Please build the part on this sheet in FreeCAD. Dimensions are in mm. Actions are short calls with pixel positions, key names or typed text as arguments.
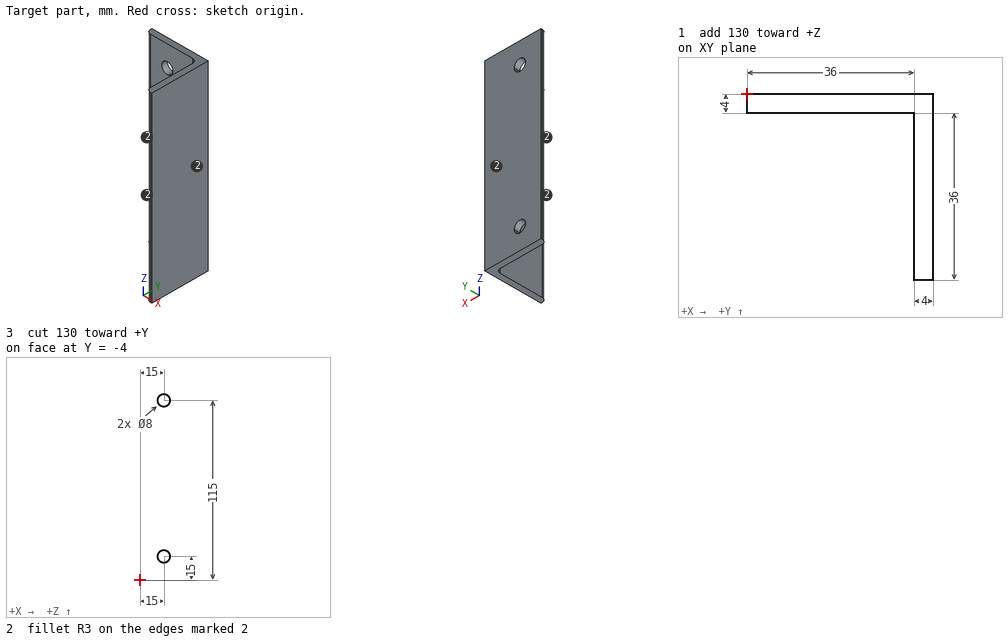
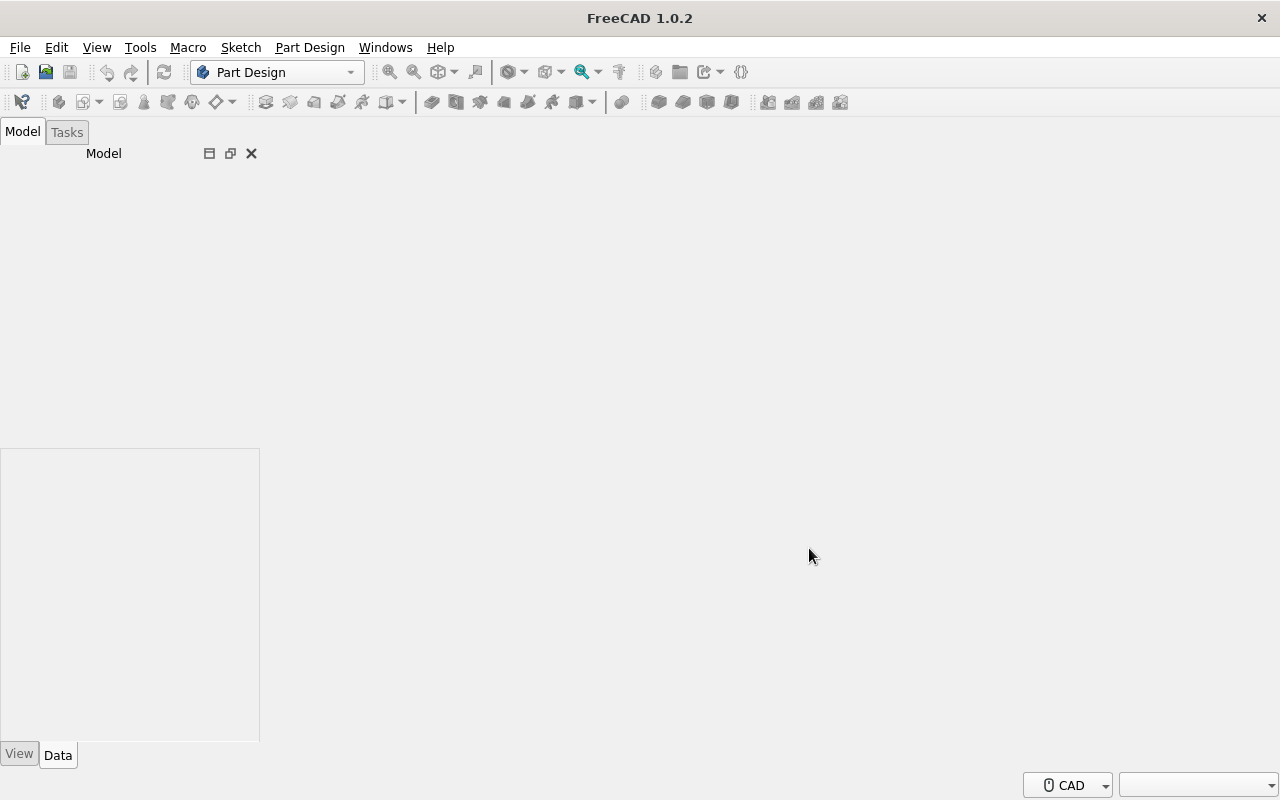
click(22, 72)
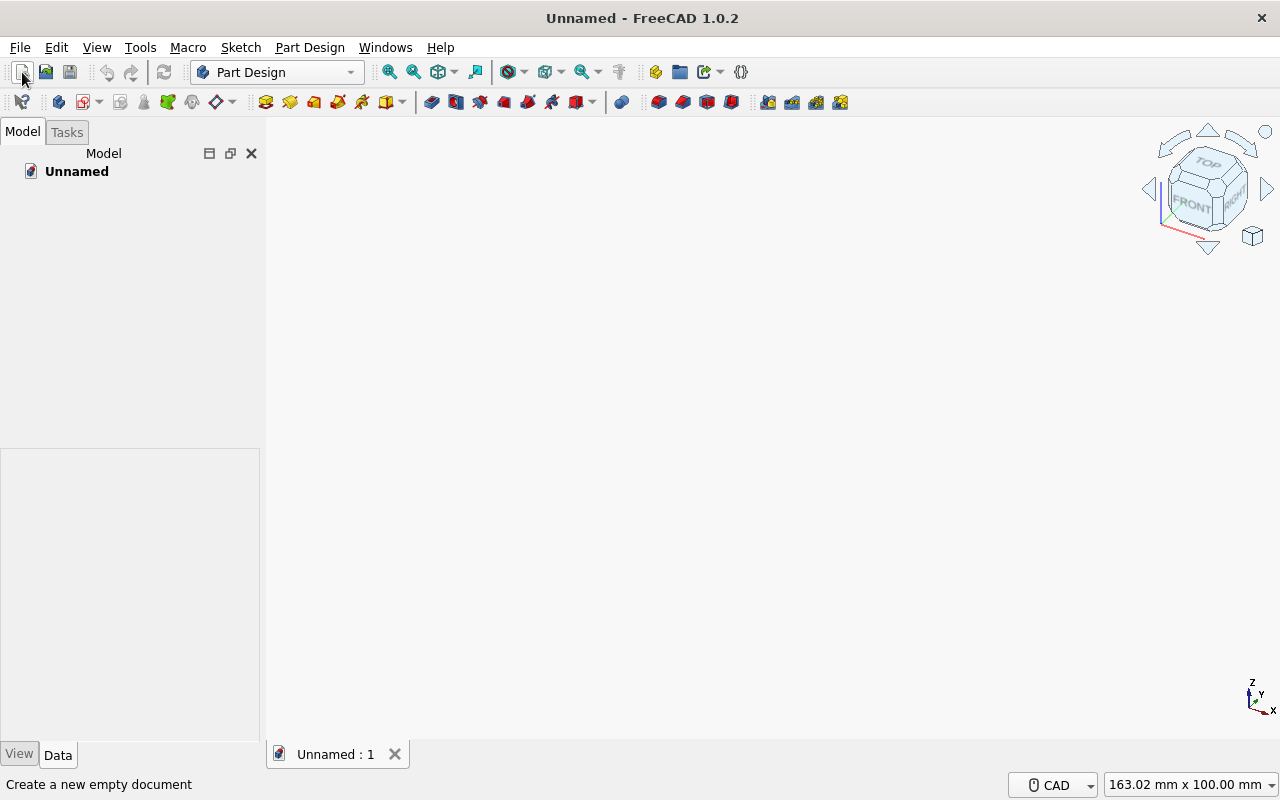
click(84, 102)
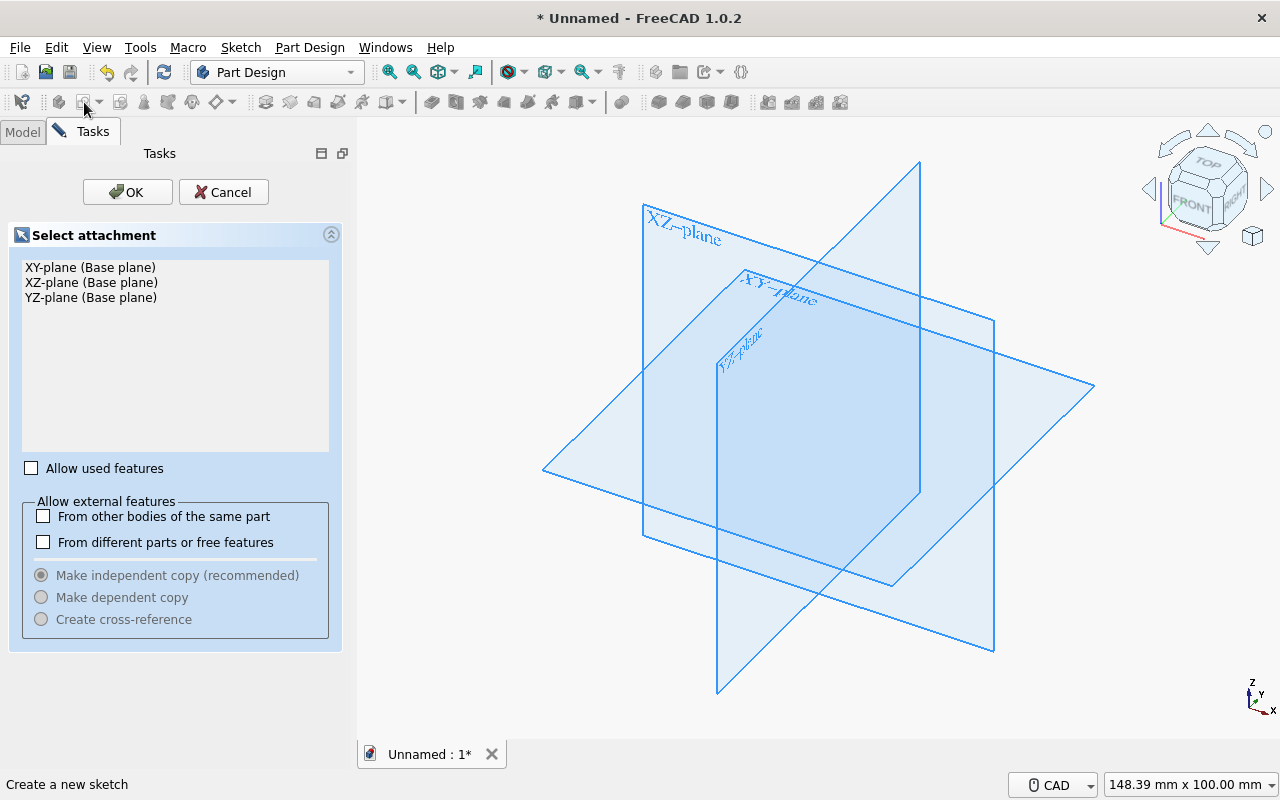
click(82, 268)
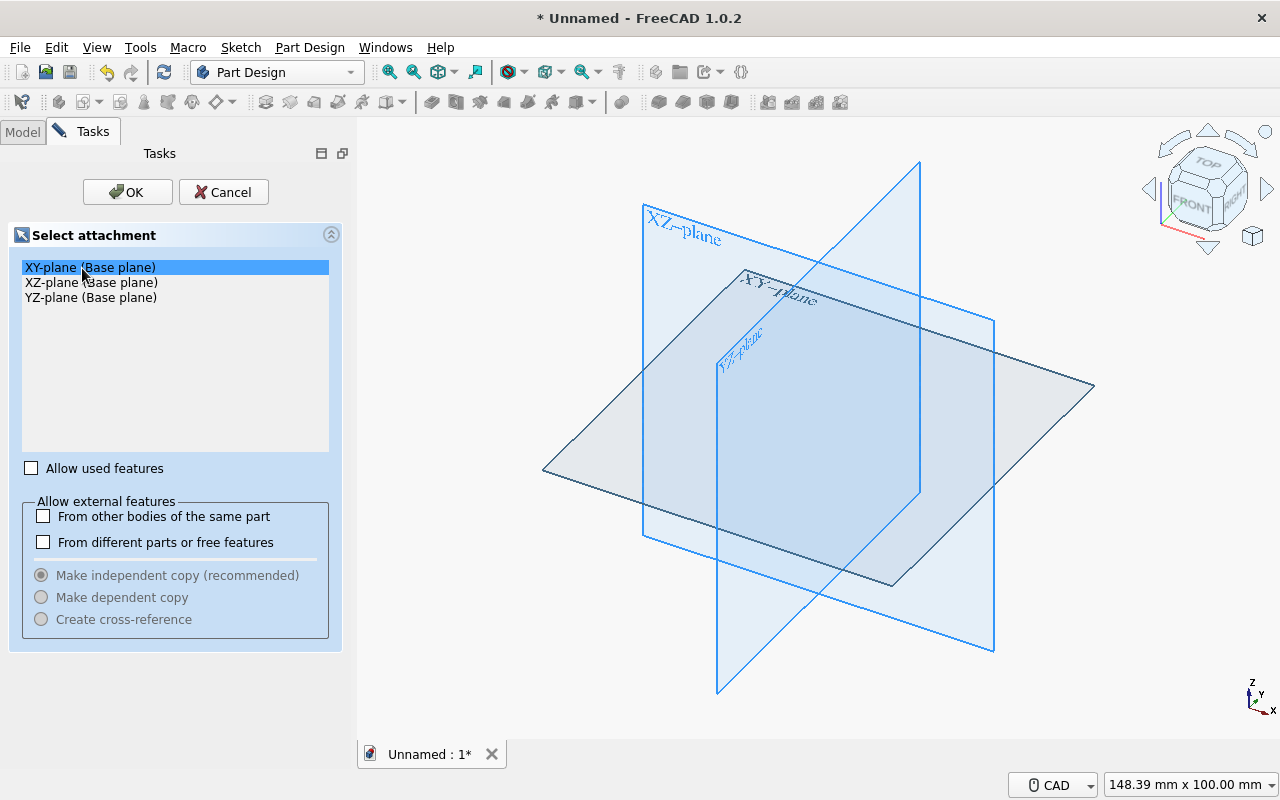
click(128, 192)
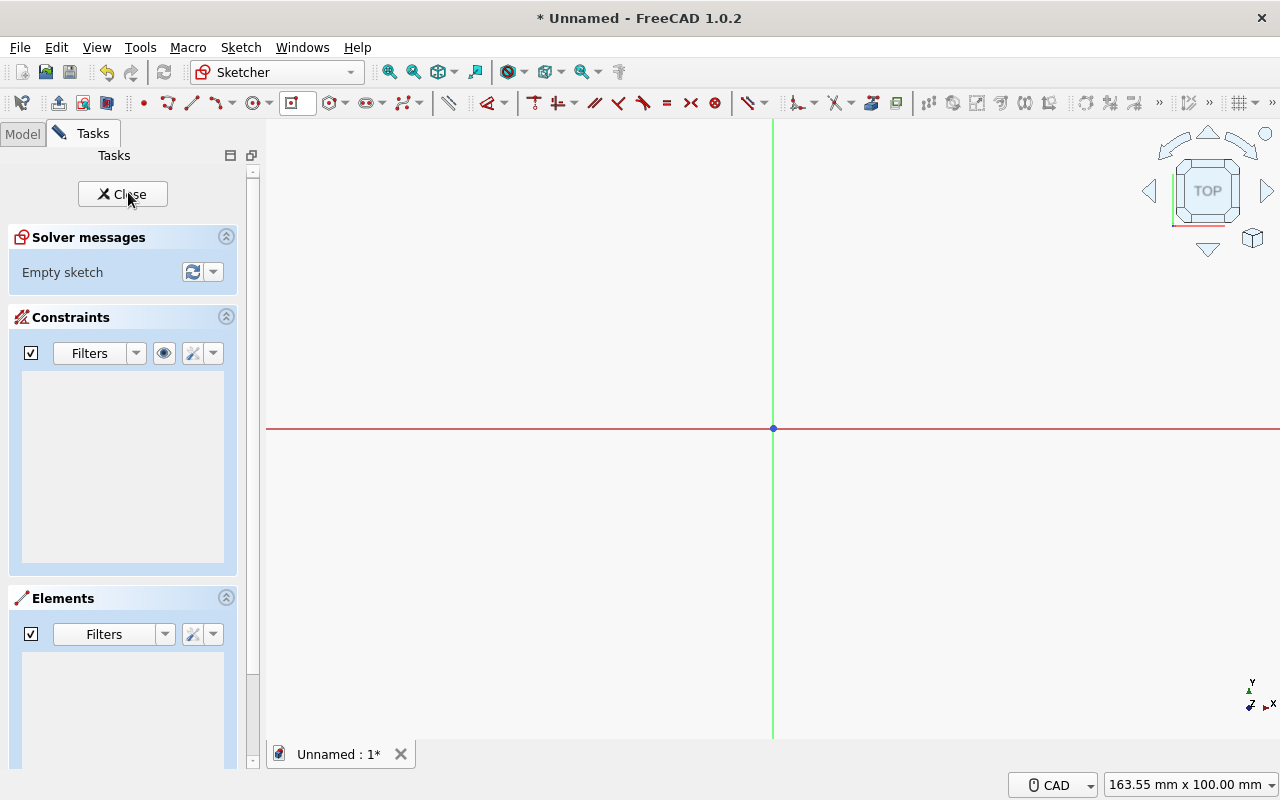
scroll(1115, 711, up, 2)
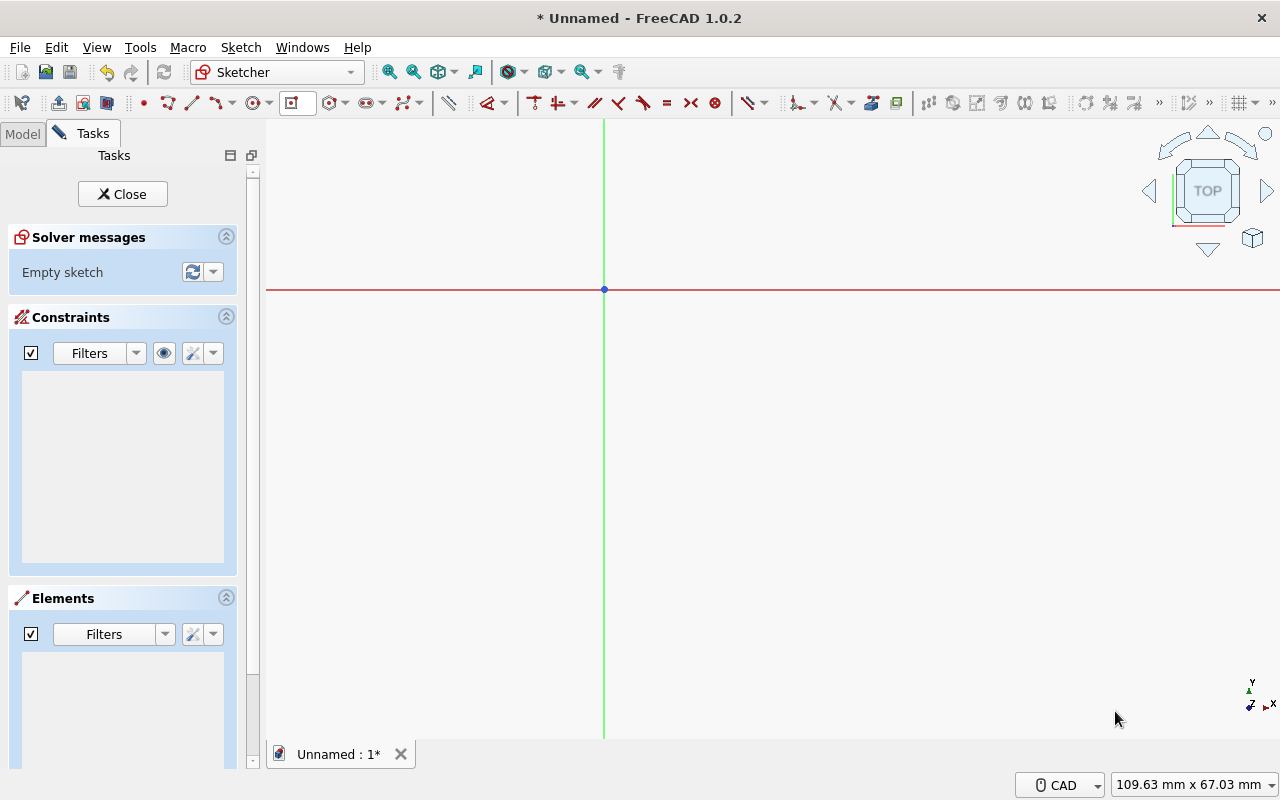
click(168, 104)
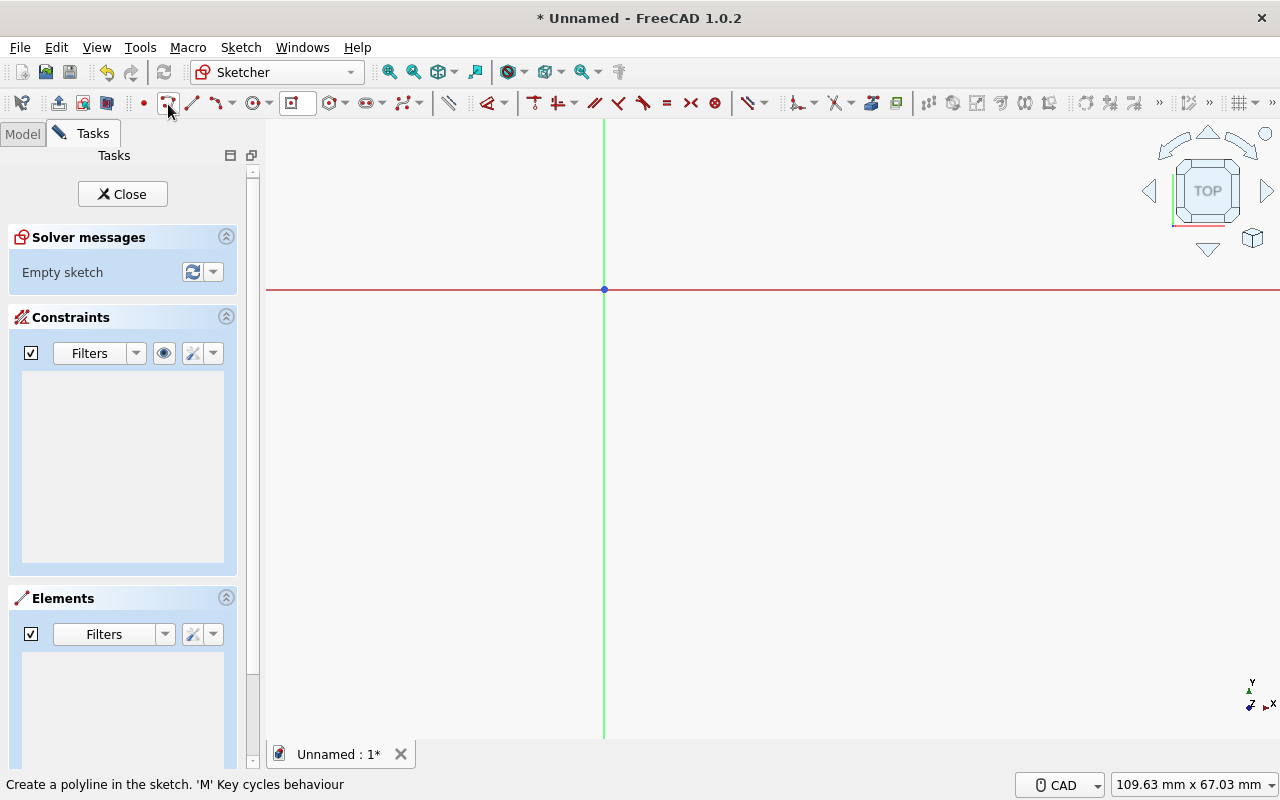
click(604, 290)
click(613, 327)
click(937, 327)
click(937, 660)
click(974, 660)
click(974, 299)
click(604, 290)
key(Escape)
key(Escape)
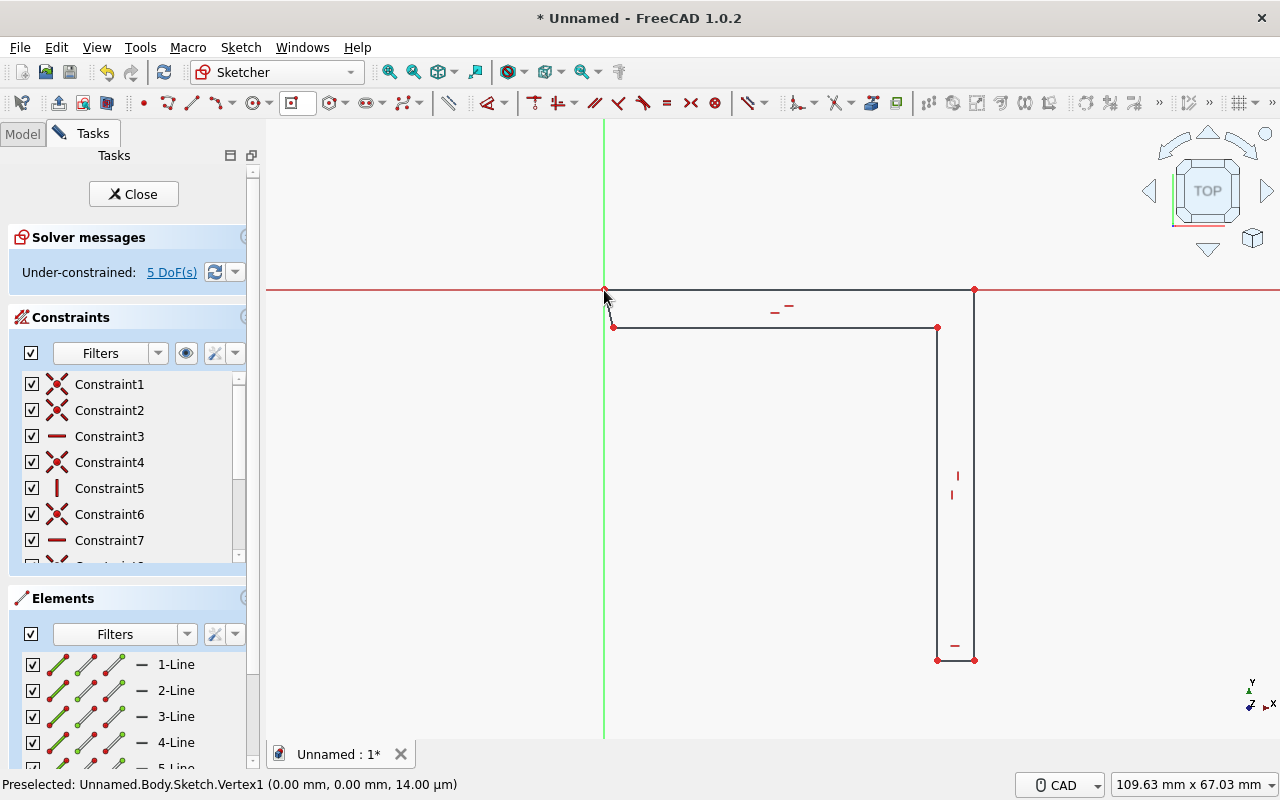
click(607, 301)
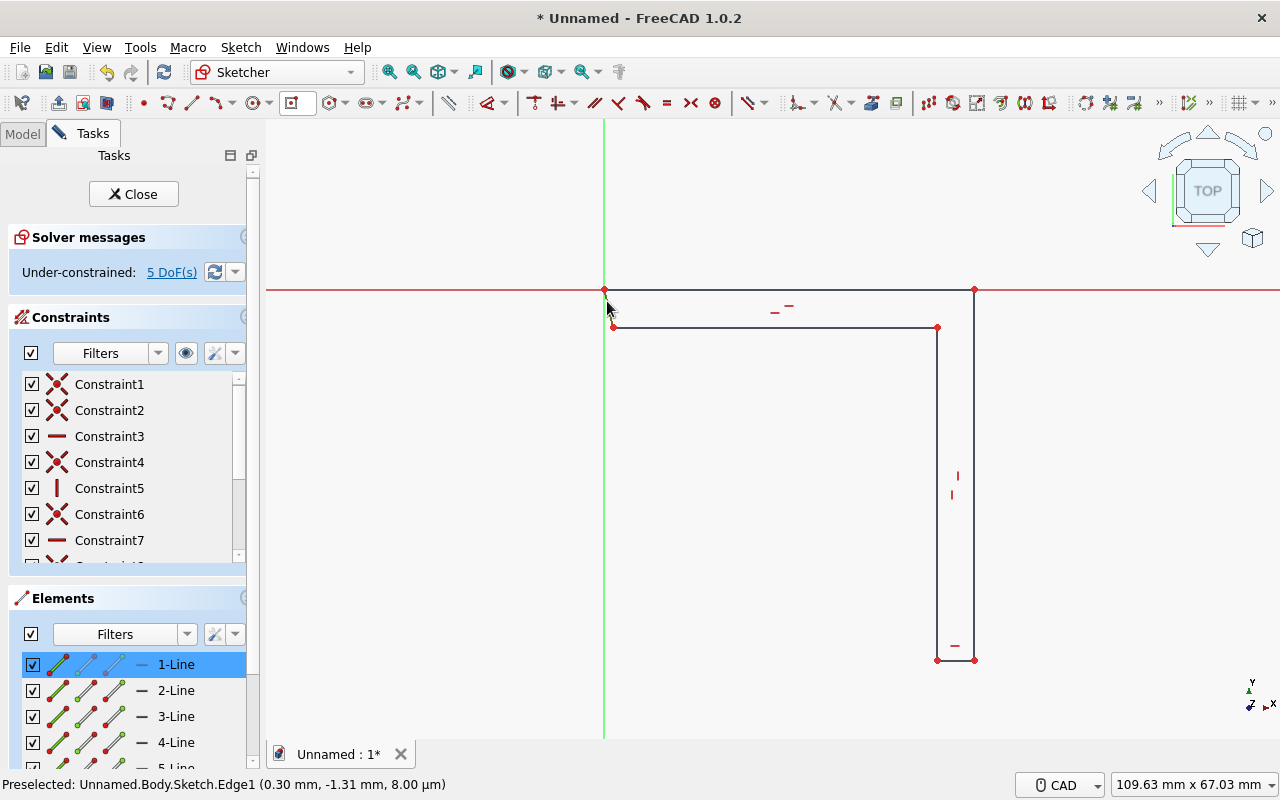
key(v)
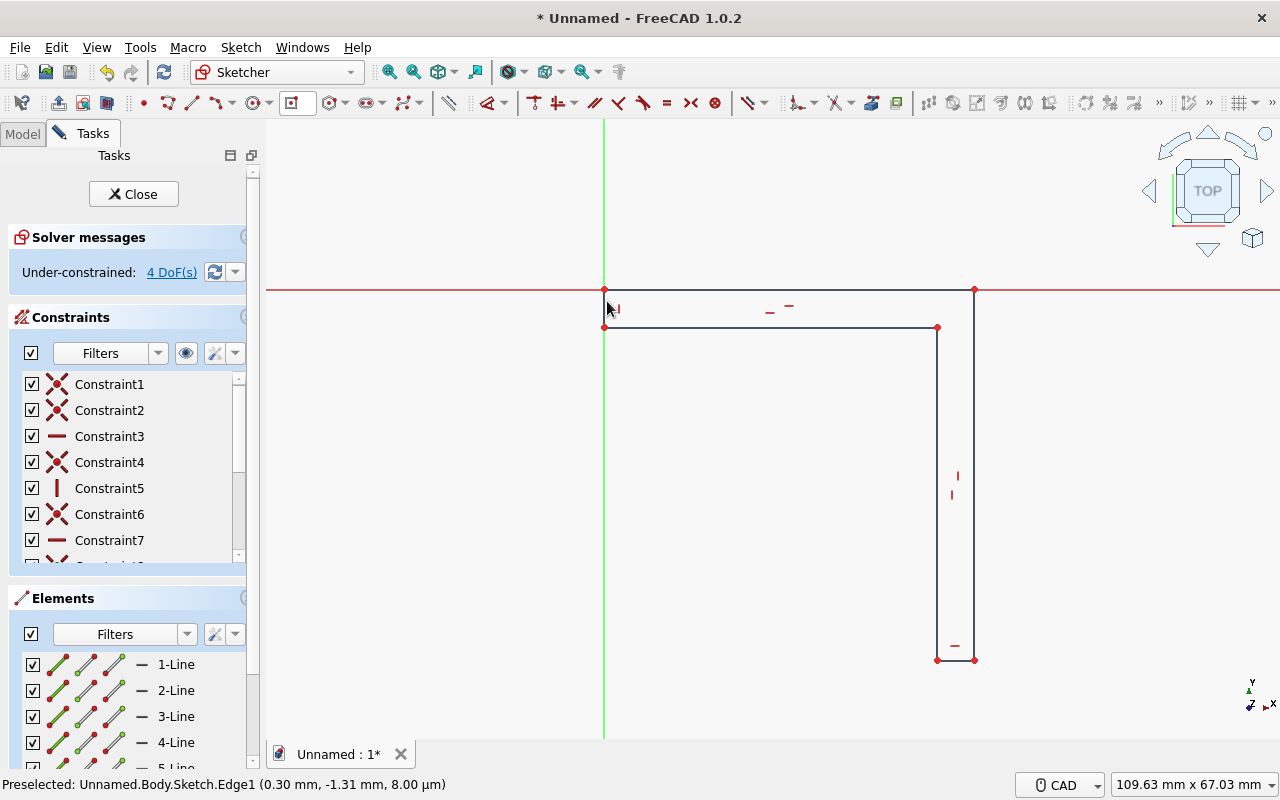
click(488, 104)